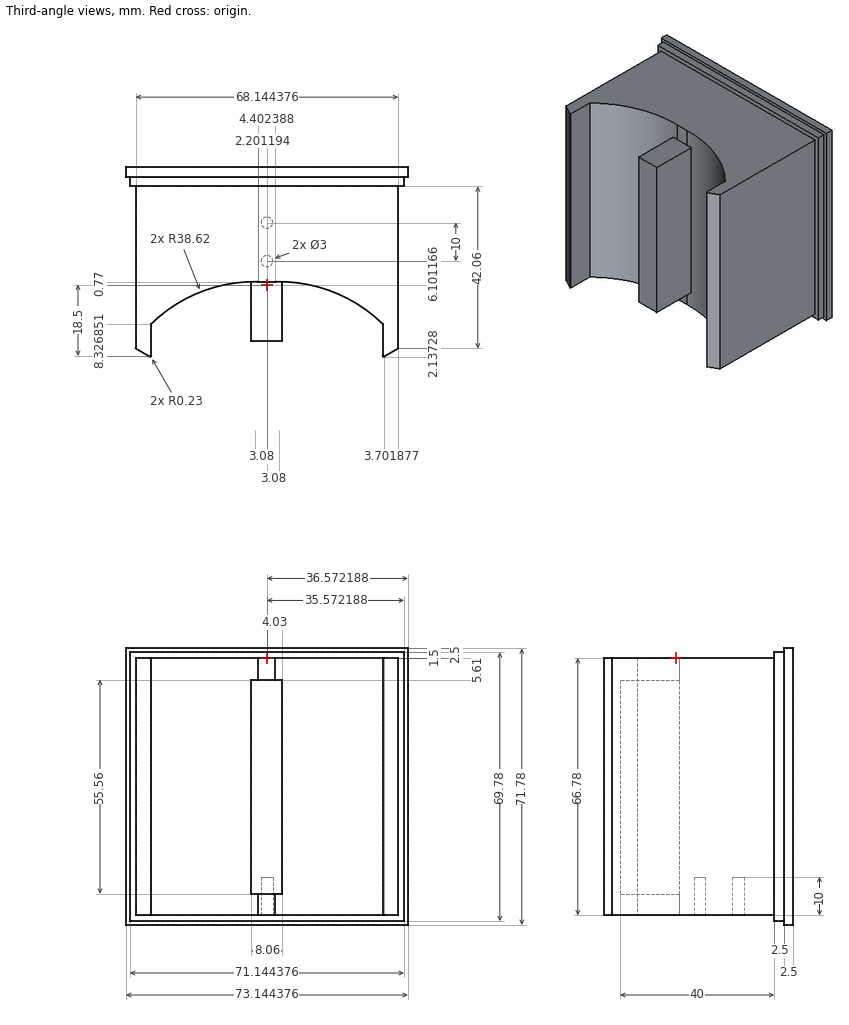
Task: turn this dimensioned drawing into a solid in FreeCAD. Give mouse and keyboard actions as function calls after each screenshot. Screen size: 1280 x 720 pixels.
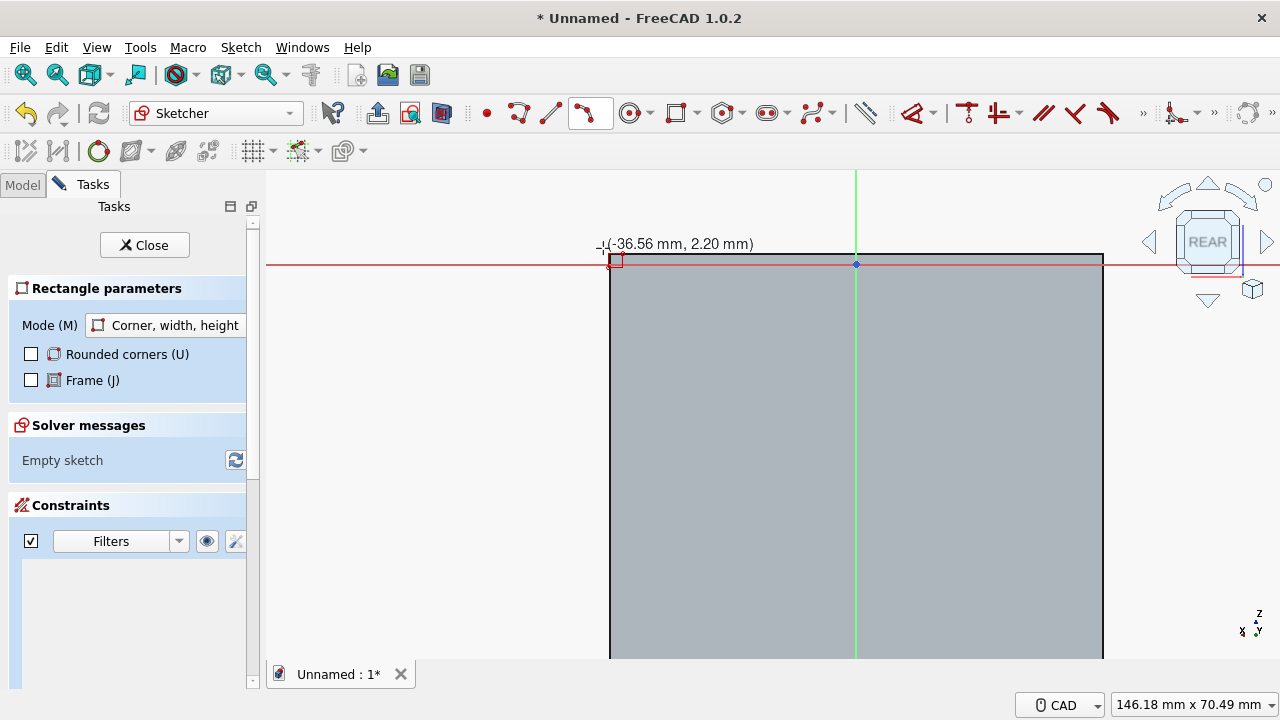
click(603, 247)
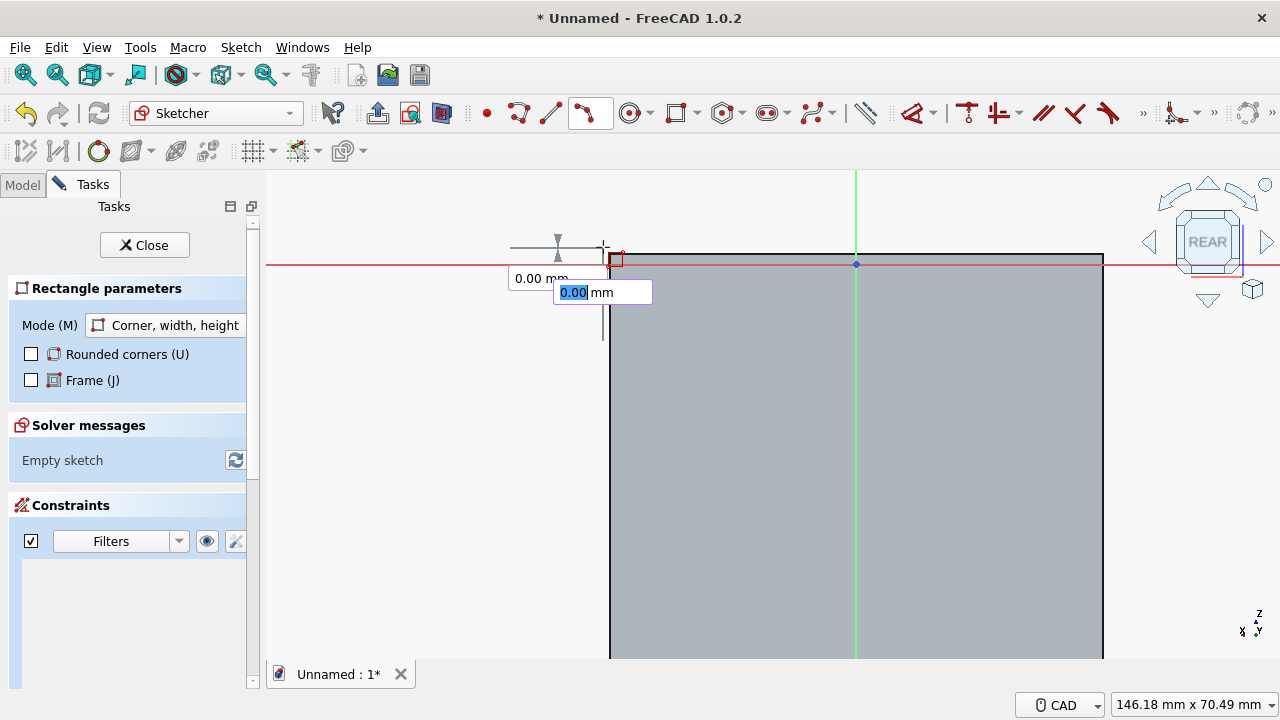
scroll(396, 248, down, 2)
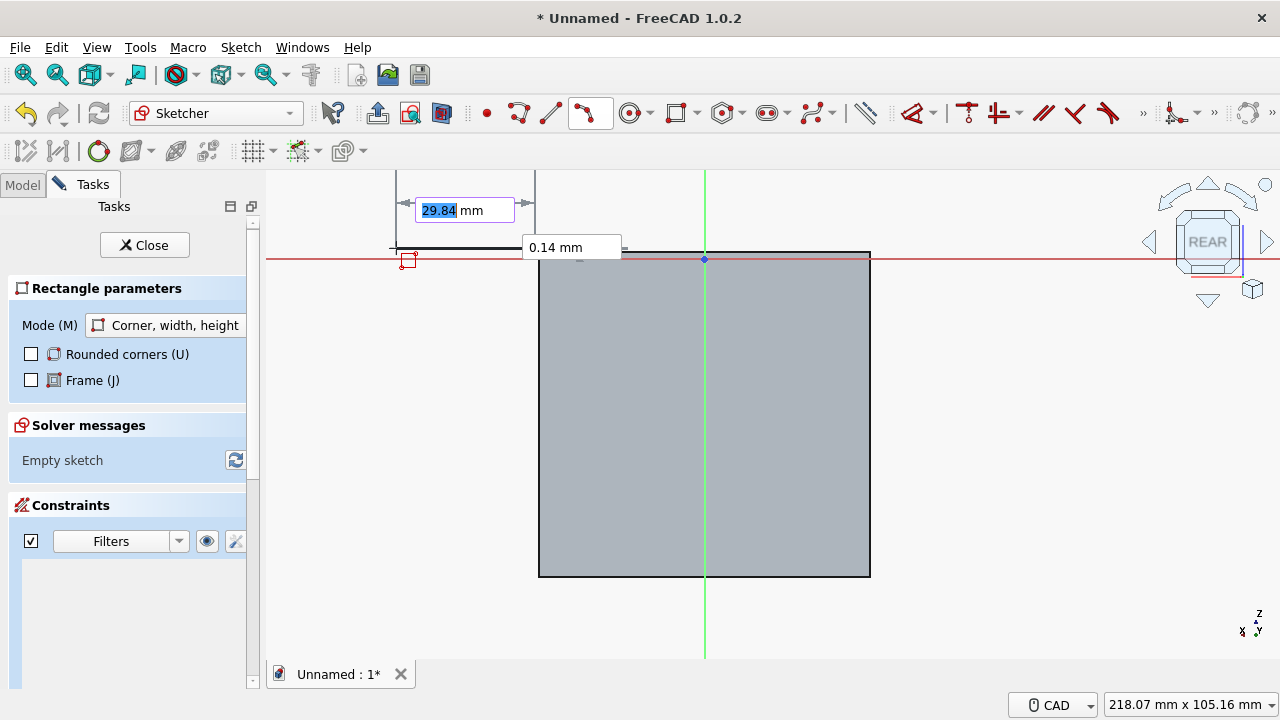
click(875, 581)
key(Escape)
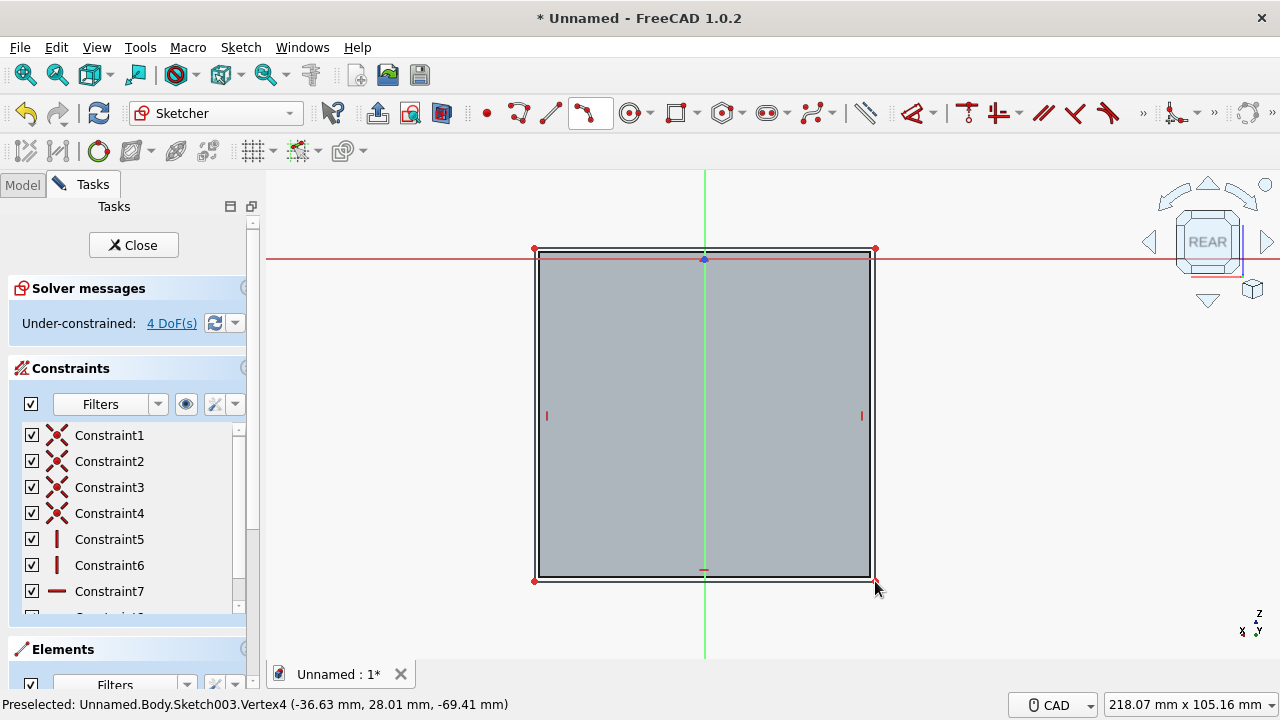
click(912, 114)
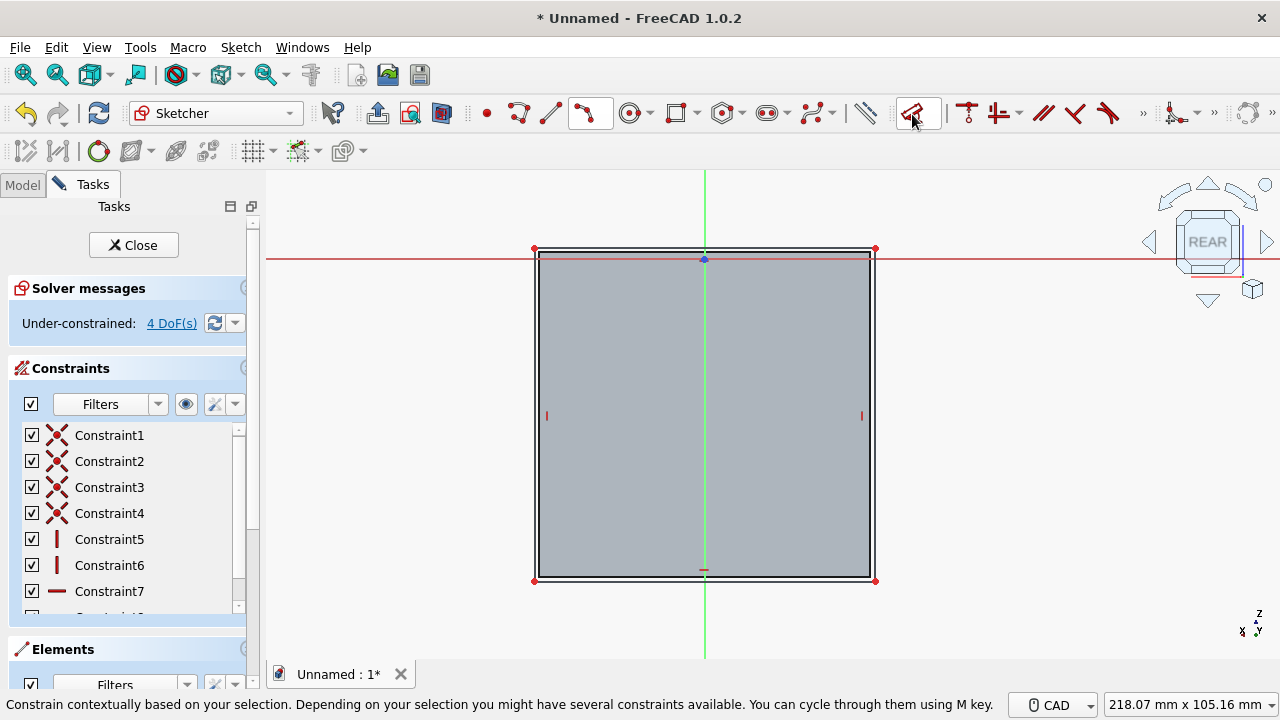
scroll(535, 248, up, 7)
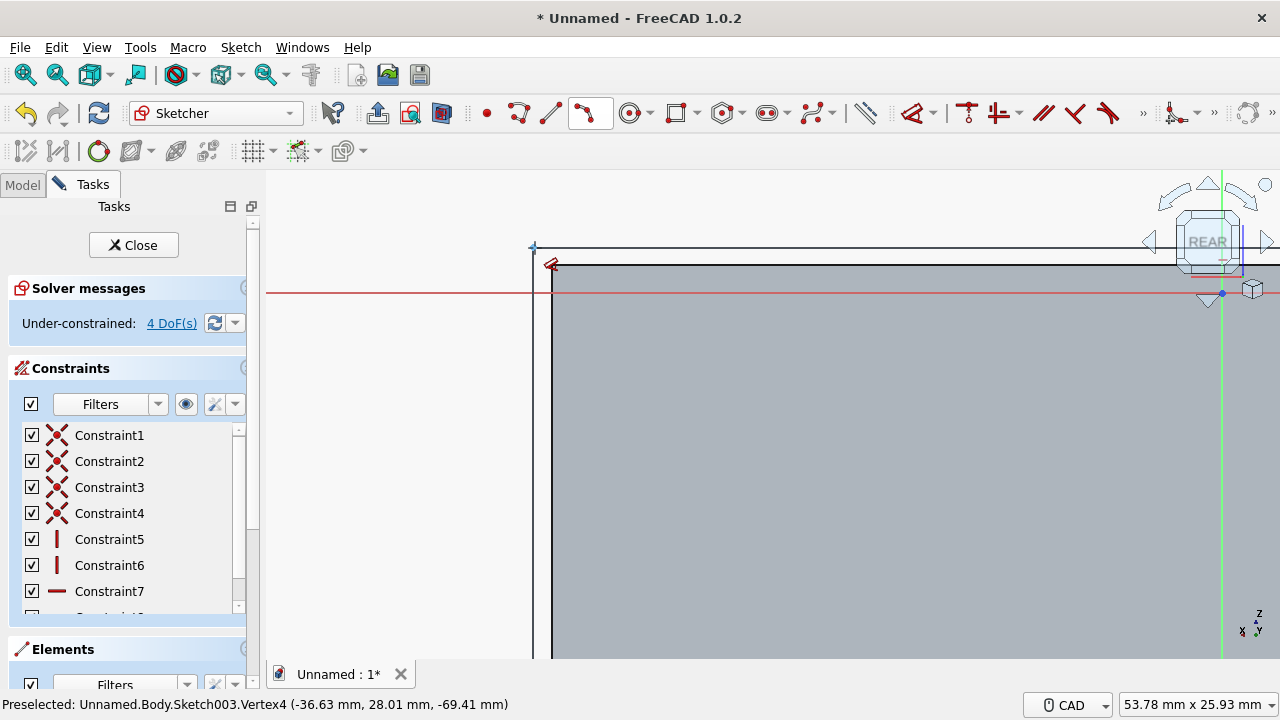
click(533, 248)
click(499, 270)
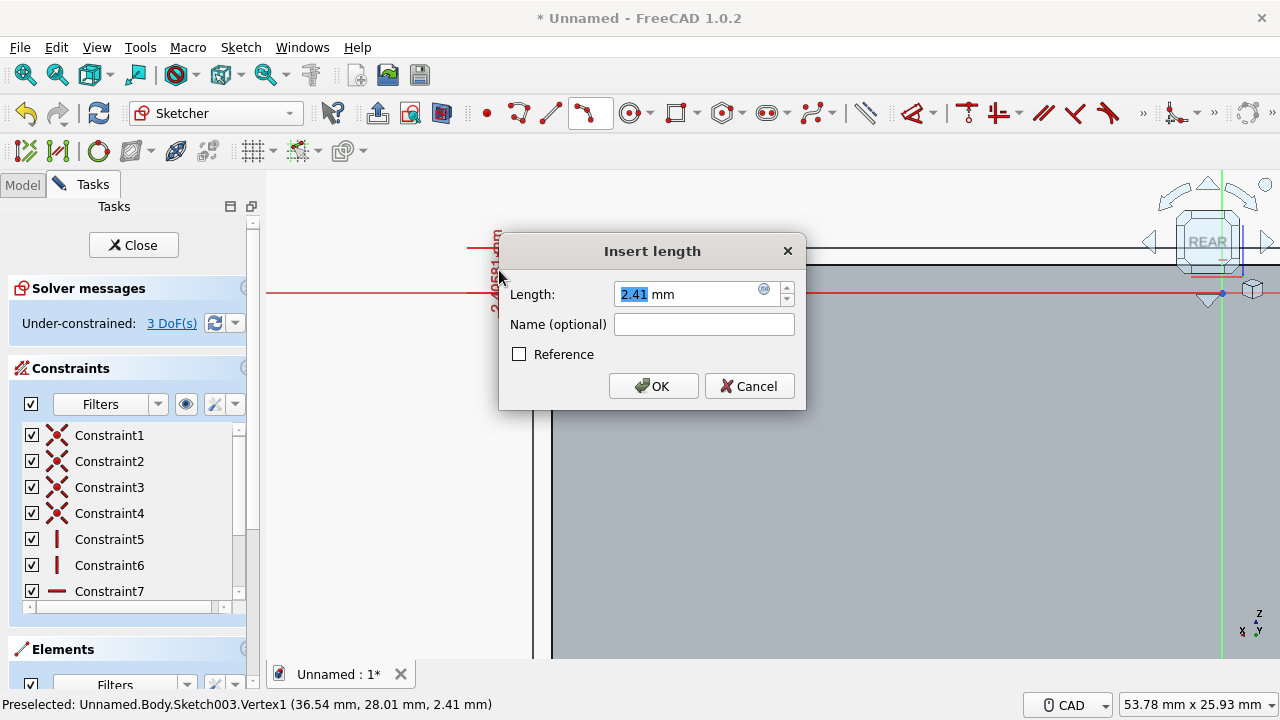
text(2.5)
key(Return)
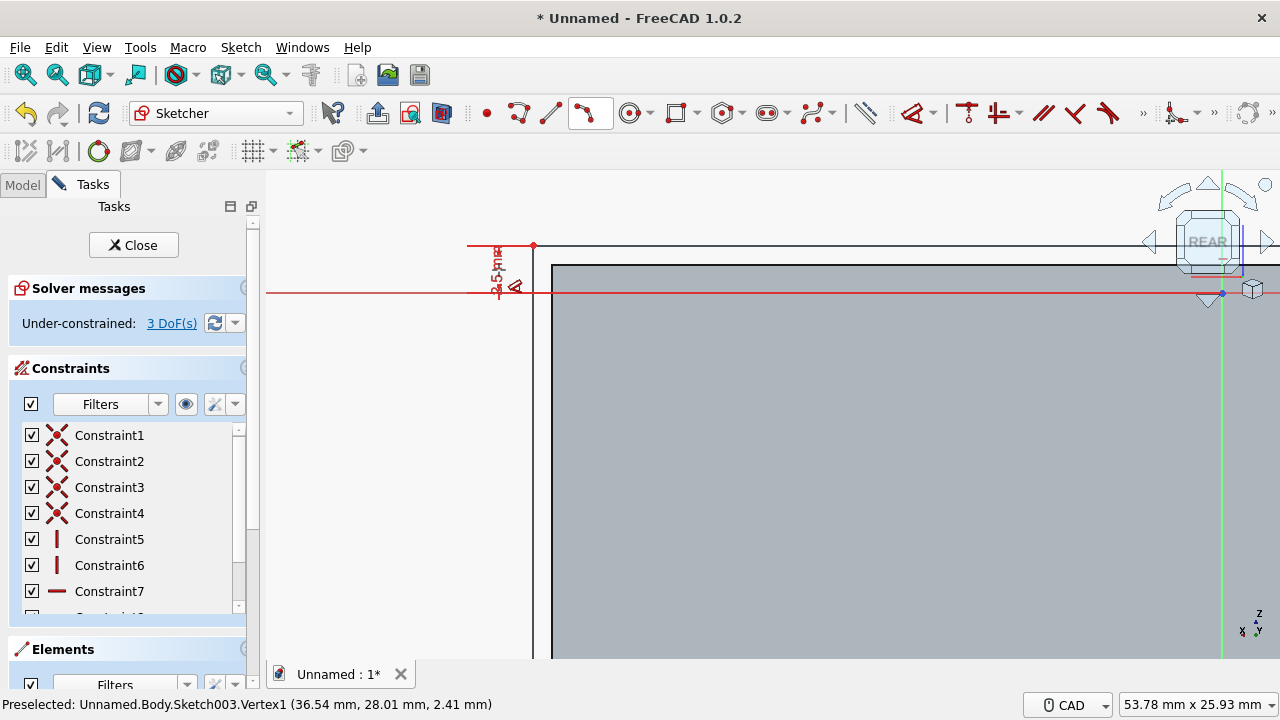
scroll(535, 248, down, 7)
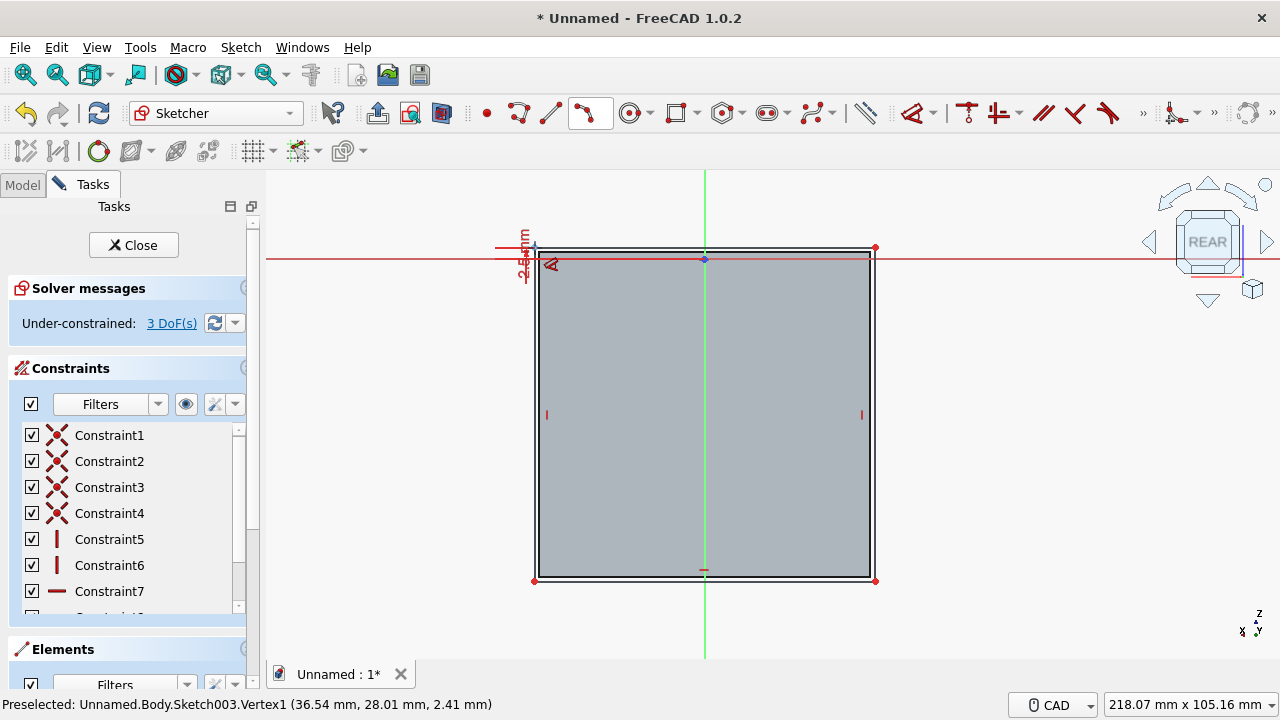
click(535, 314)
click(501, 415)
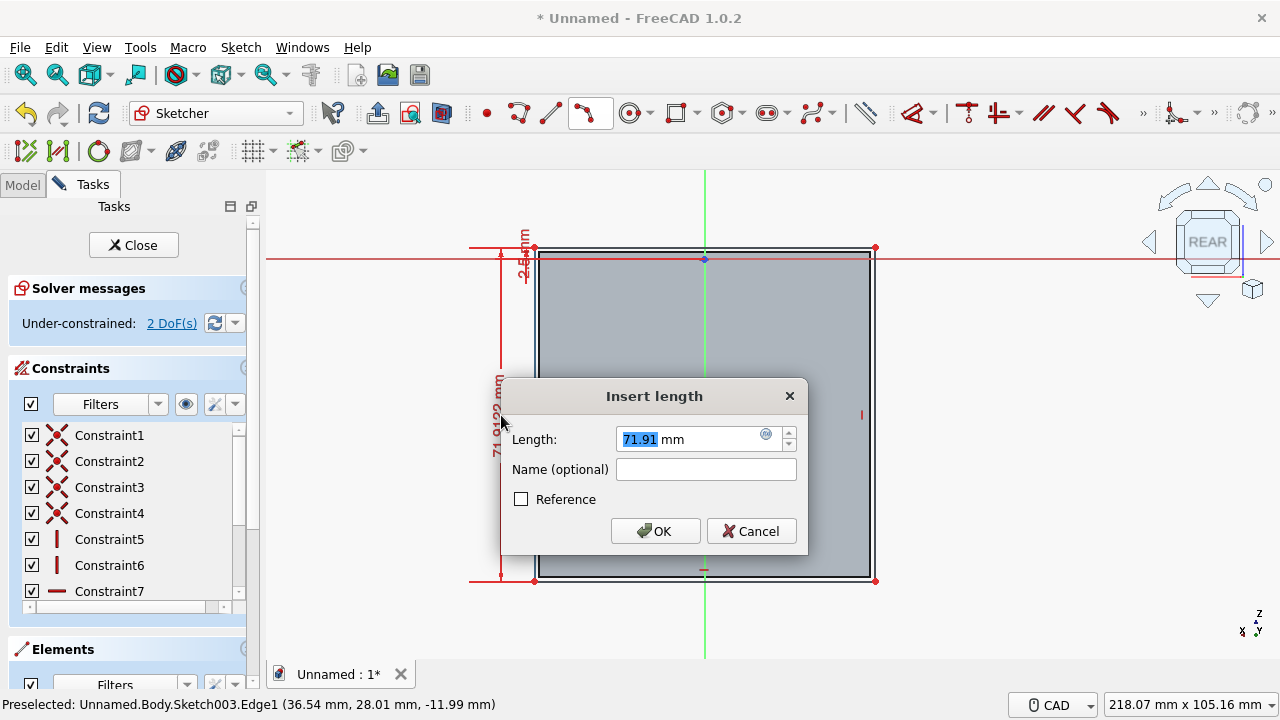
text(71.78)
key(Return)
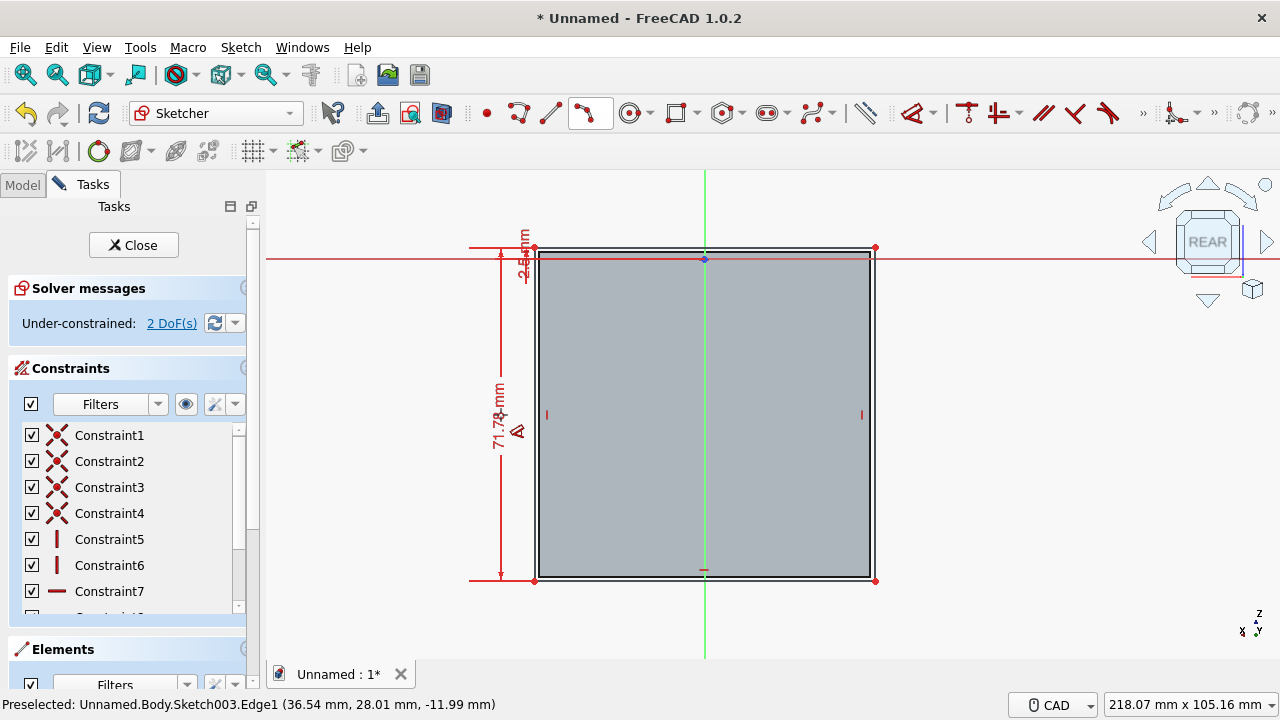
click(637, 581)
click(627, 615)